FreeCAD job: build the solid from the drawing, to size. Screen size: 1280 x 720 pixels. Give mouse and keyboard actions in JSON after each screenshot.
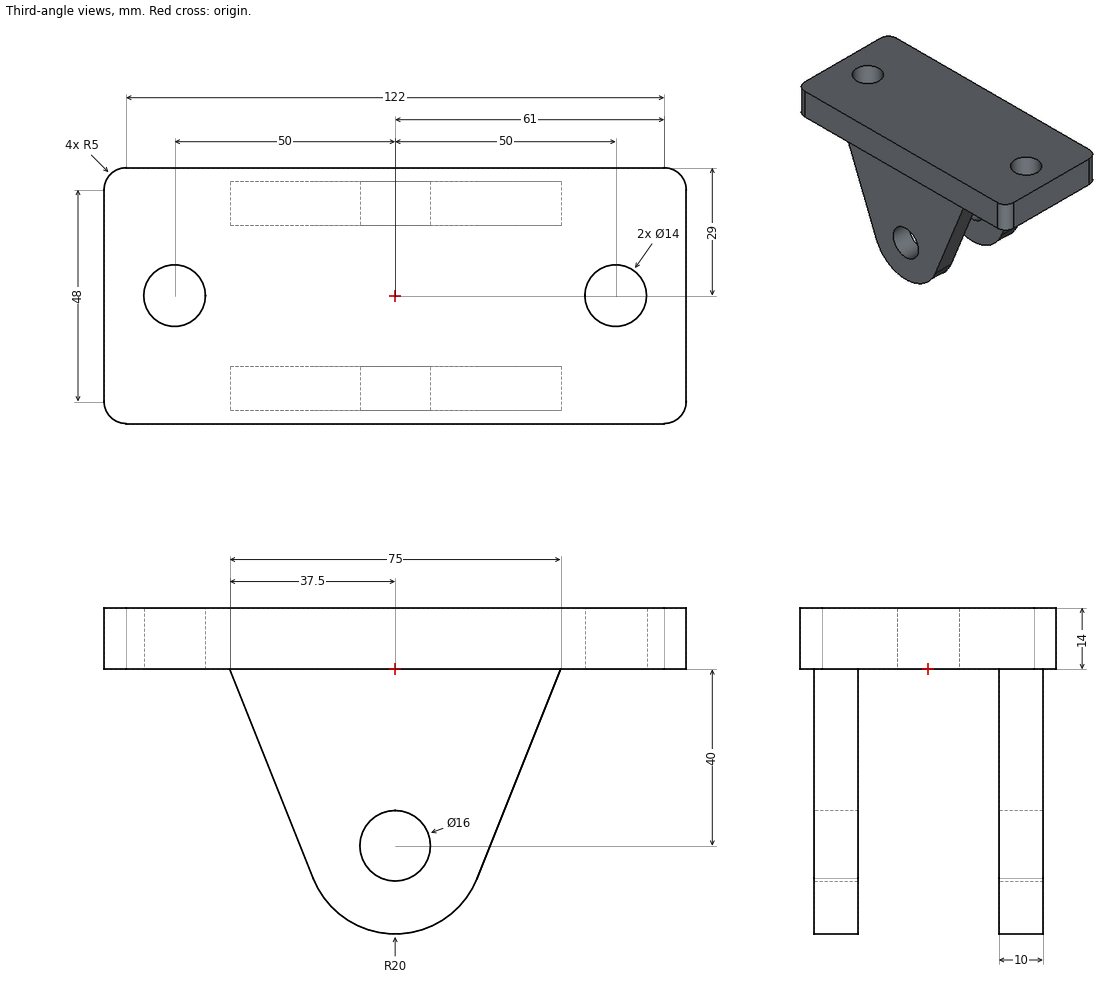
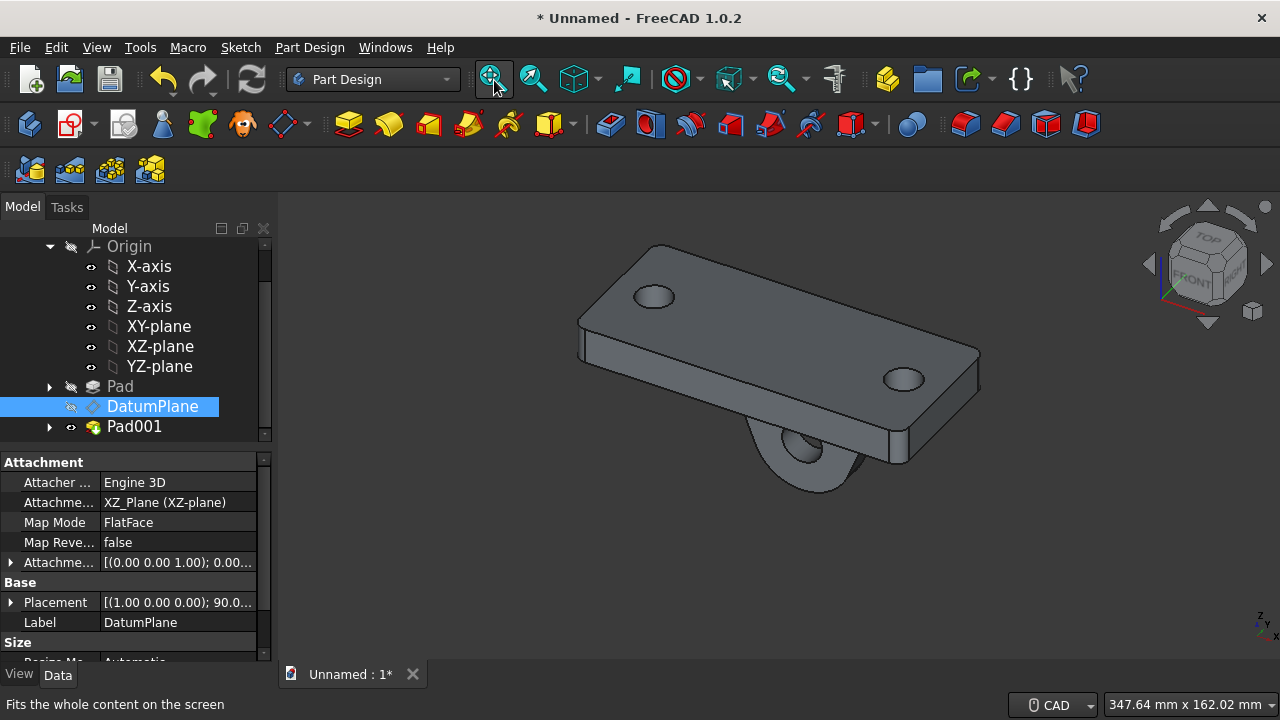
{"action": "left_click", "coordinate": [116, 427]}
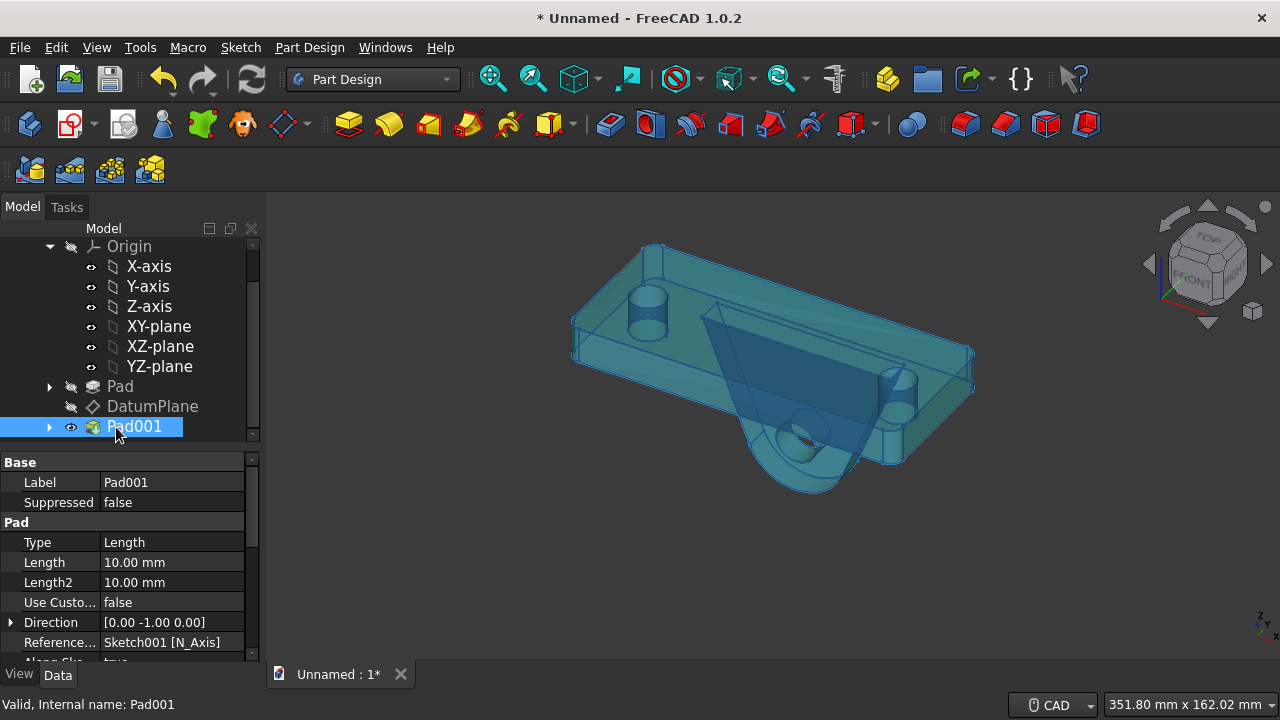
{"action": "left_click", "coordinate": [30, 170]}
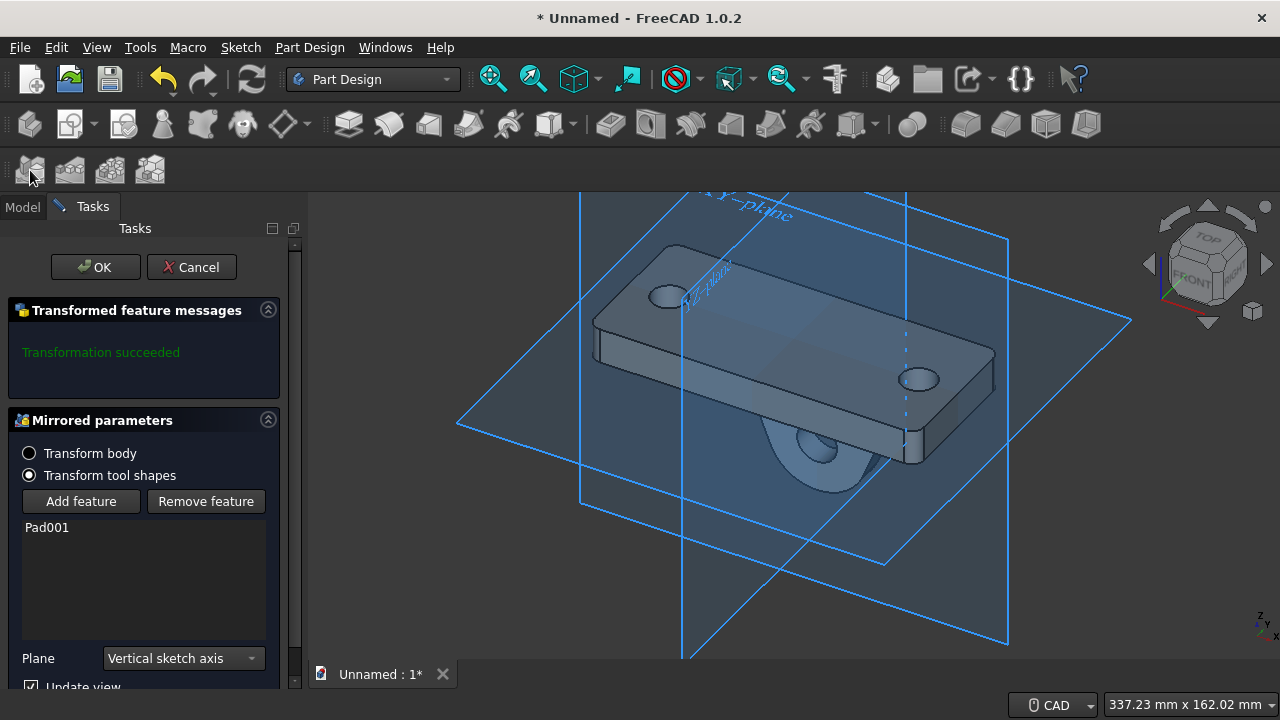
{"action": "left_click", "coordinate": [184, 658]}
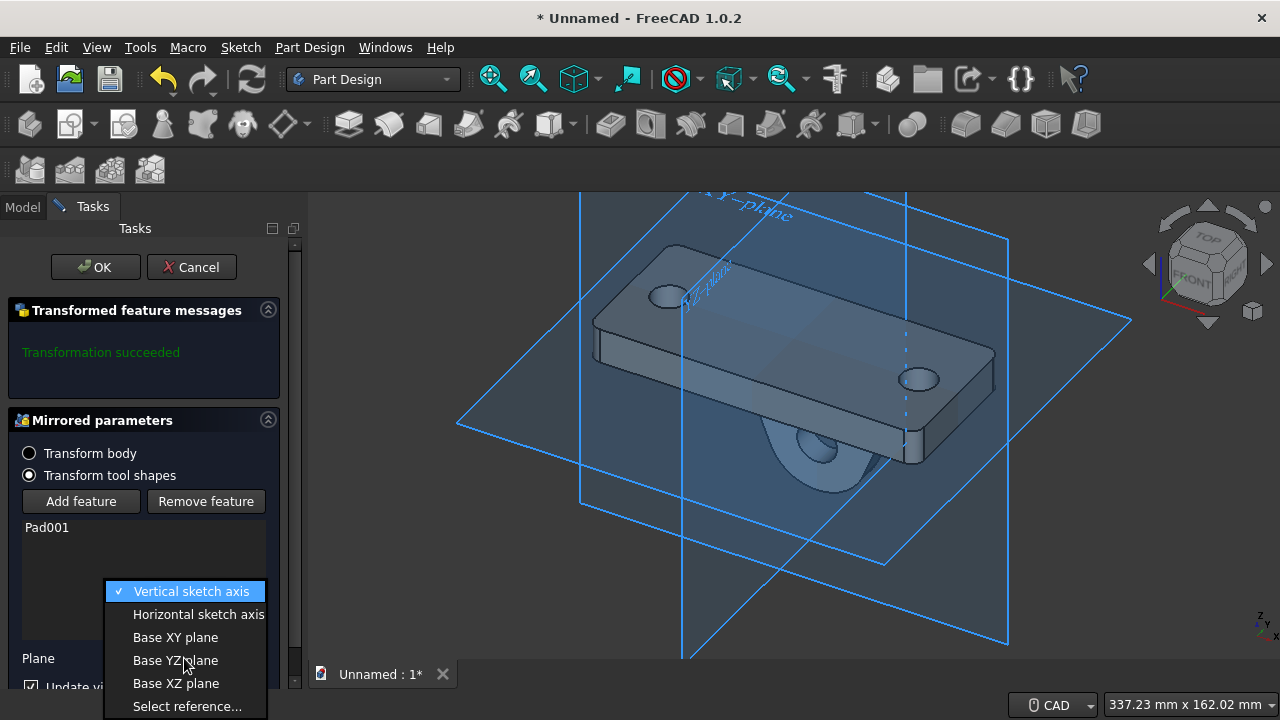
{"action": "left_click", "coordinate": [184, 684]}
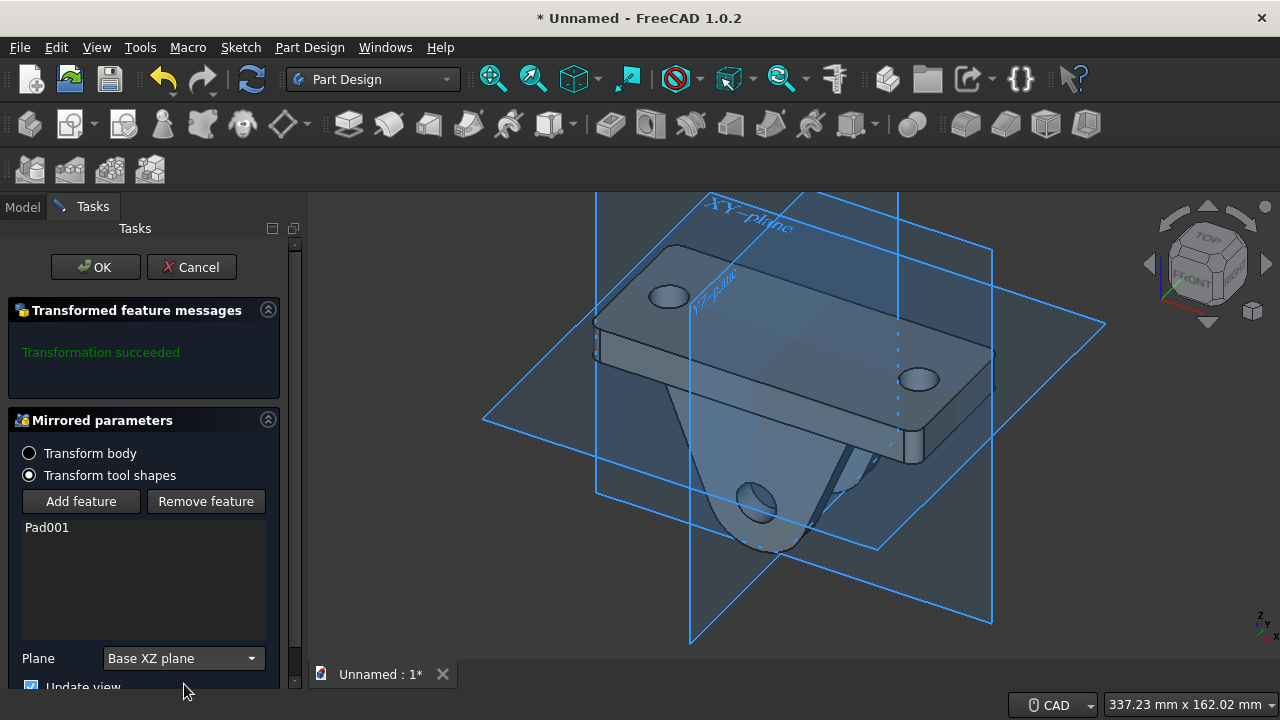
{"action": "left_click", "coordinate": [96, 267]}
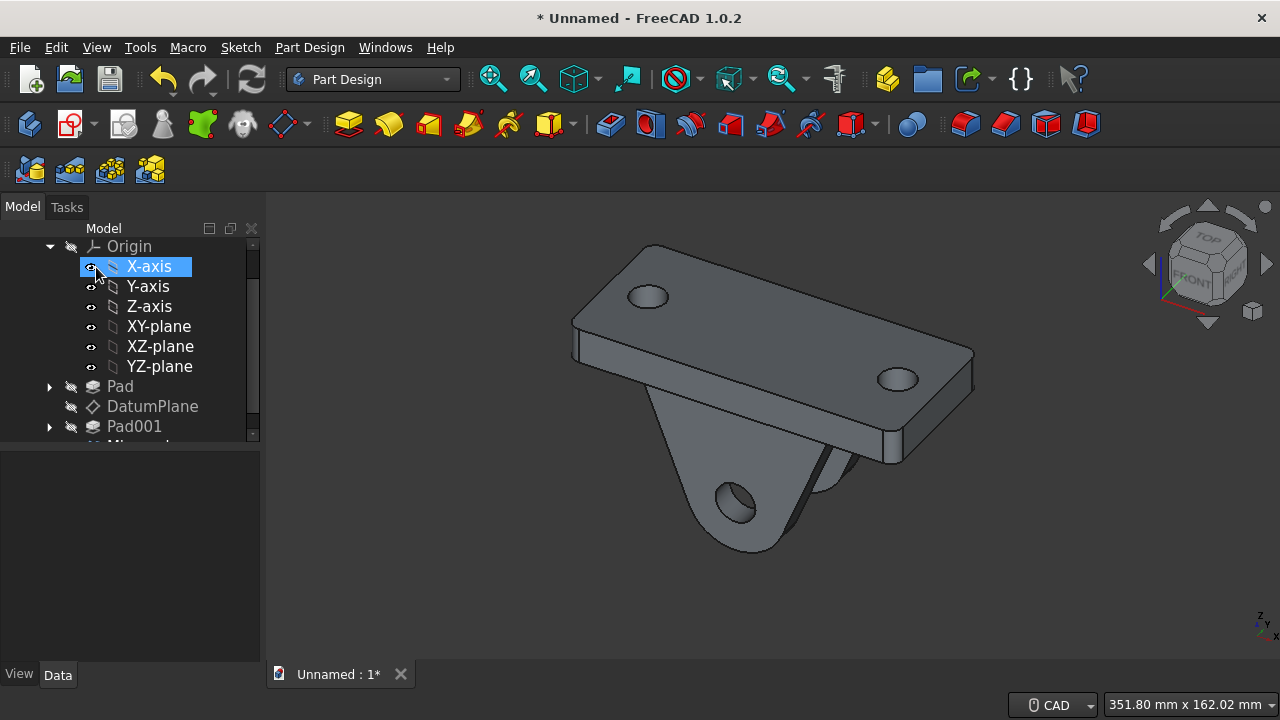
{"action": "key", "text": "0"}